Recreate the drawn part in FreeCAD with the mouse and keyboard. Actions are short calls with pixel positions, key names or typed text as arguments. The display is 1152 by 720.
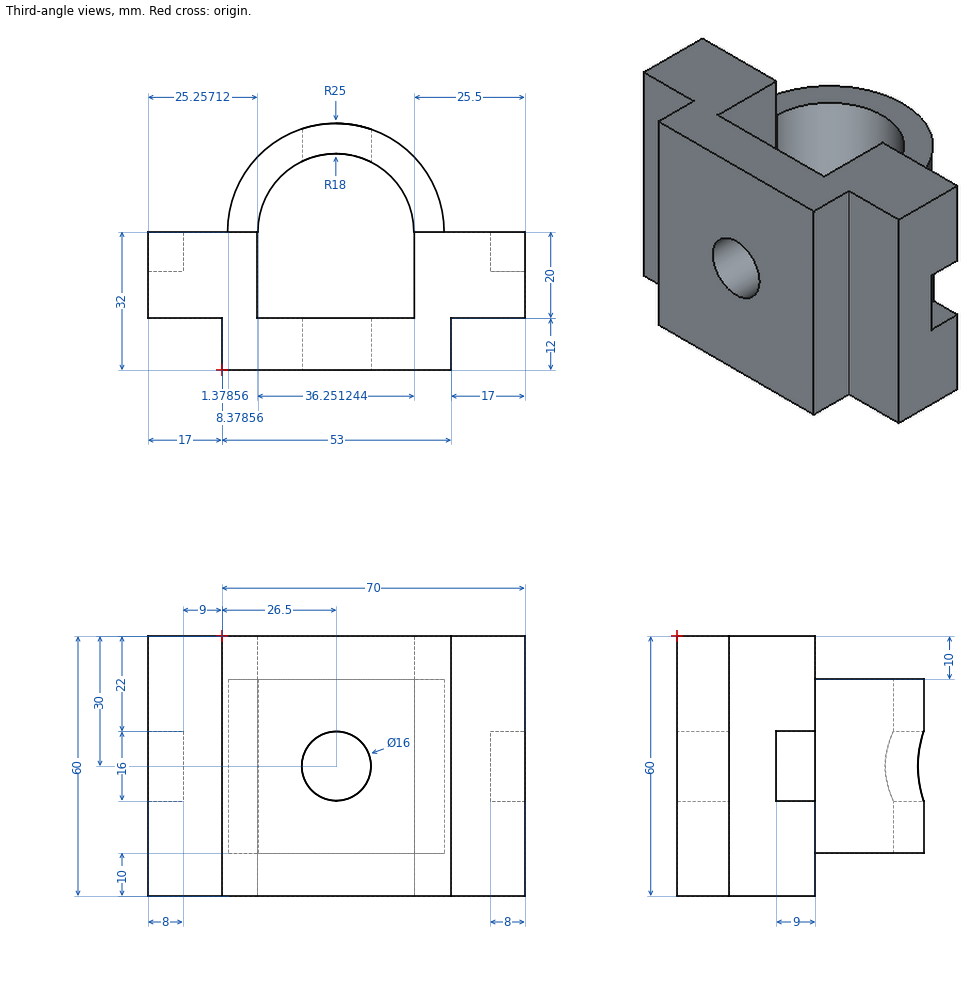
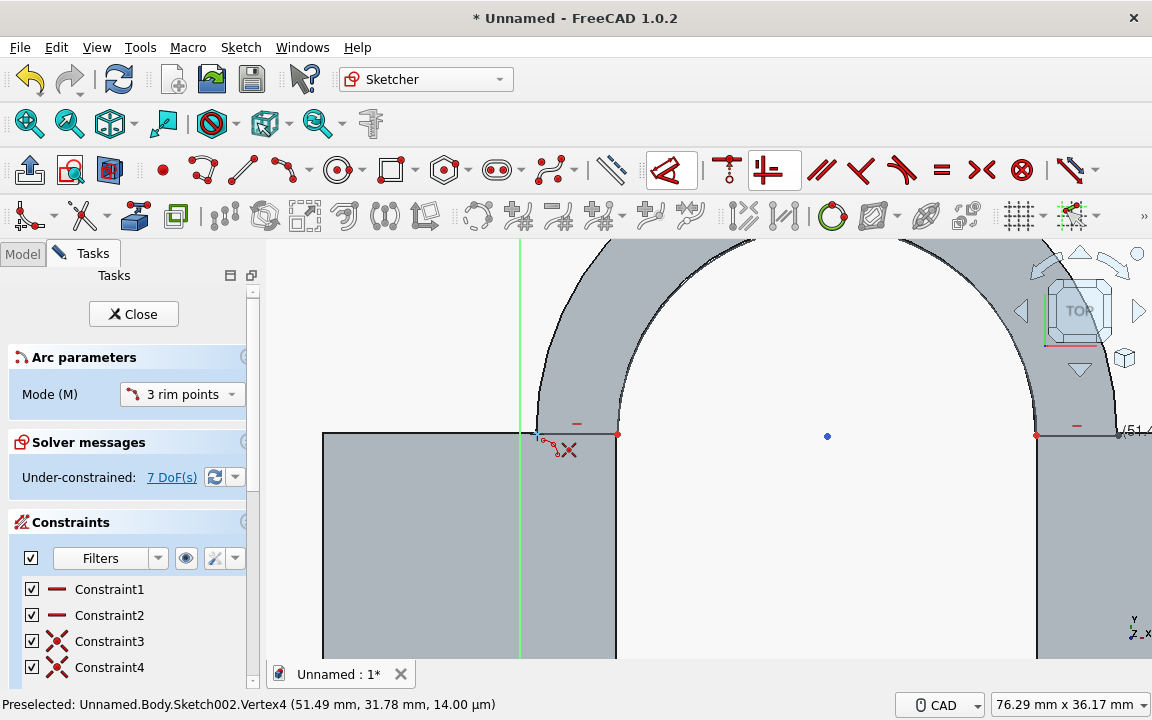
click(537, 434)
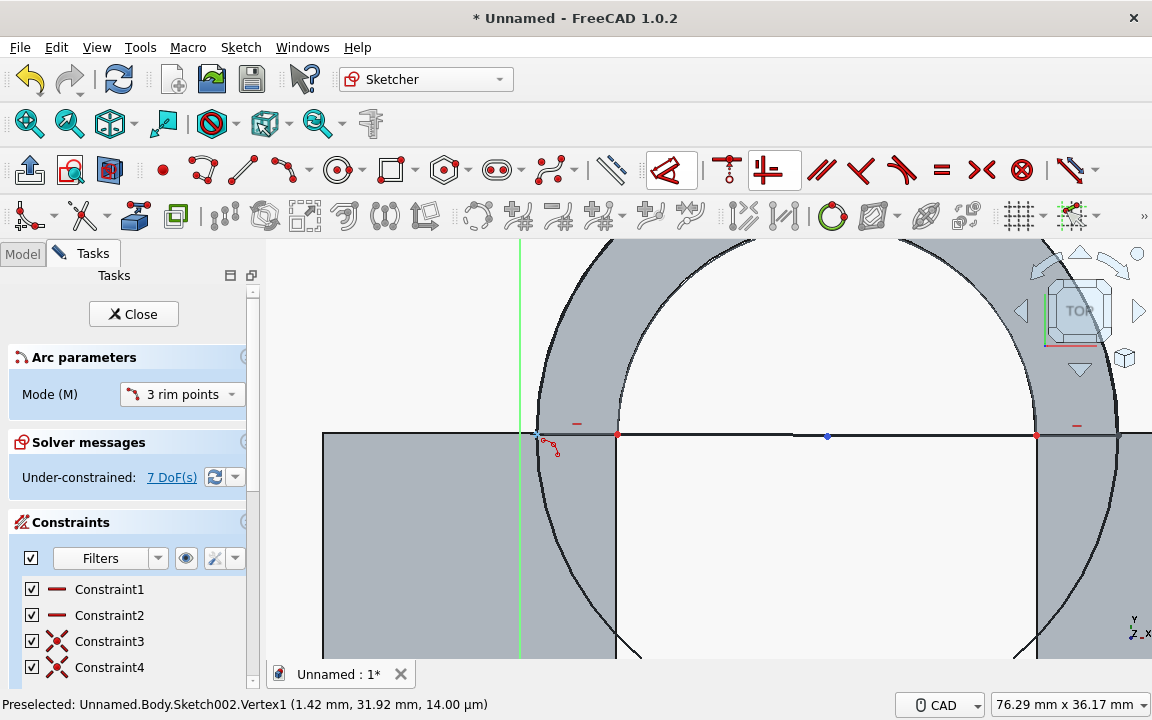
scroll(537, 434, down, 5)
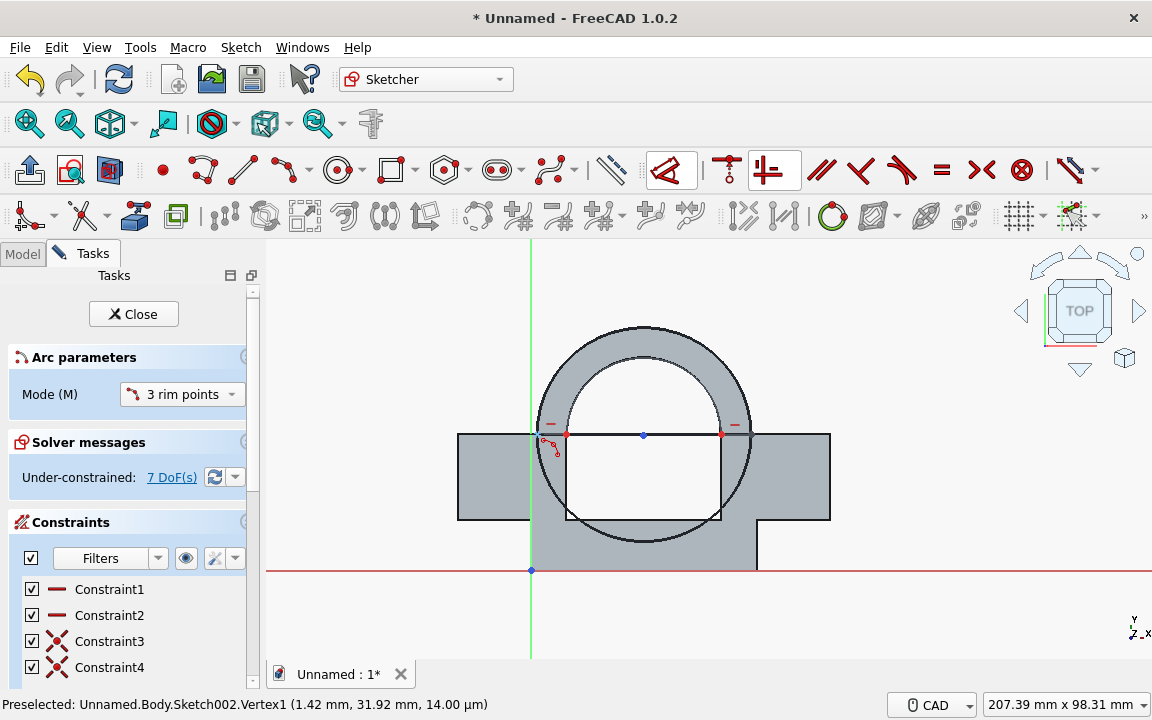
click(644, 327)
key(Escape)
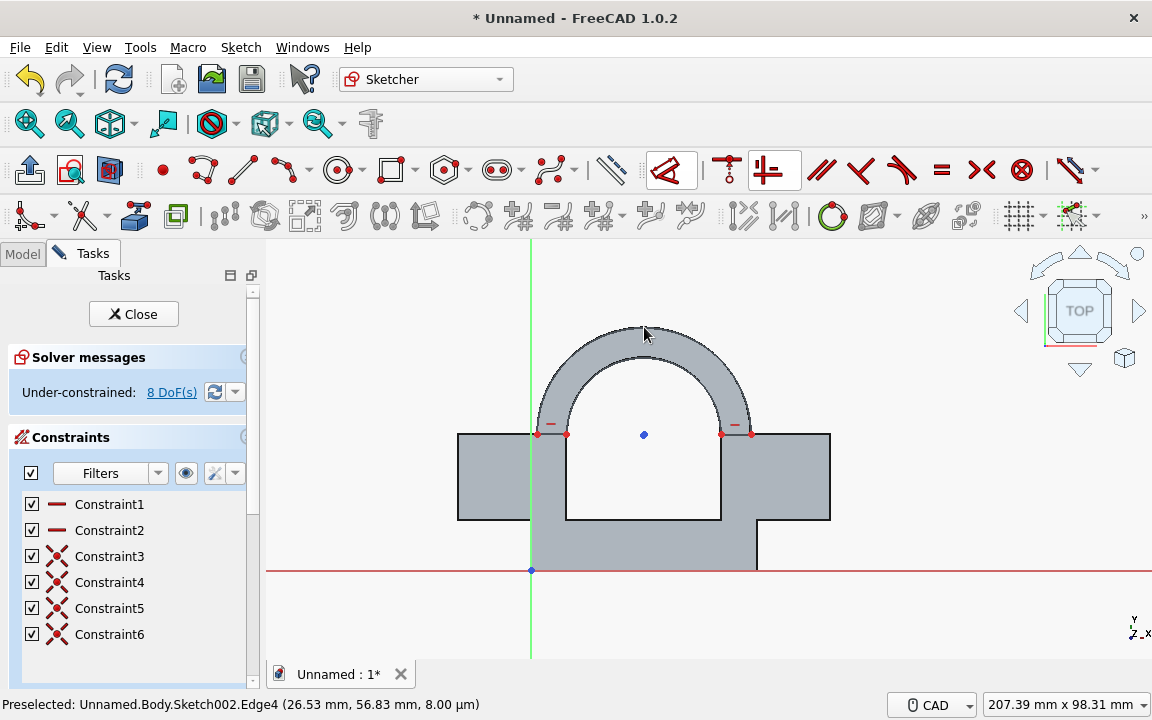
click(689, 373)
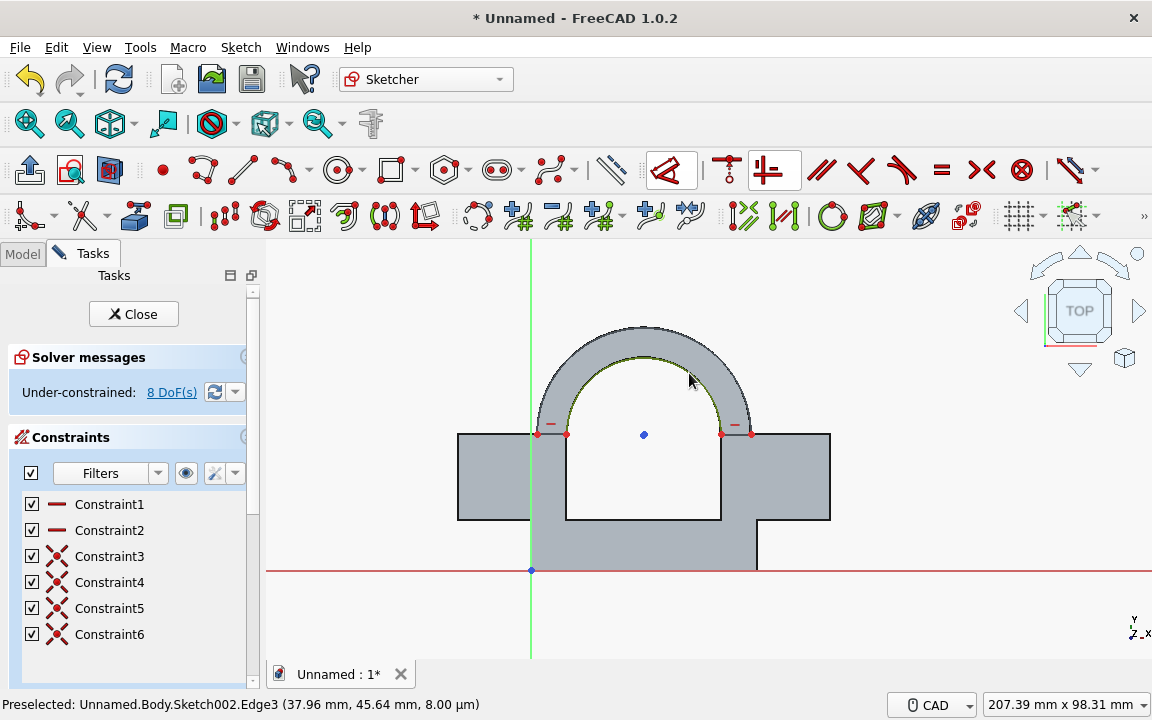
click(707, 349)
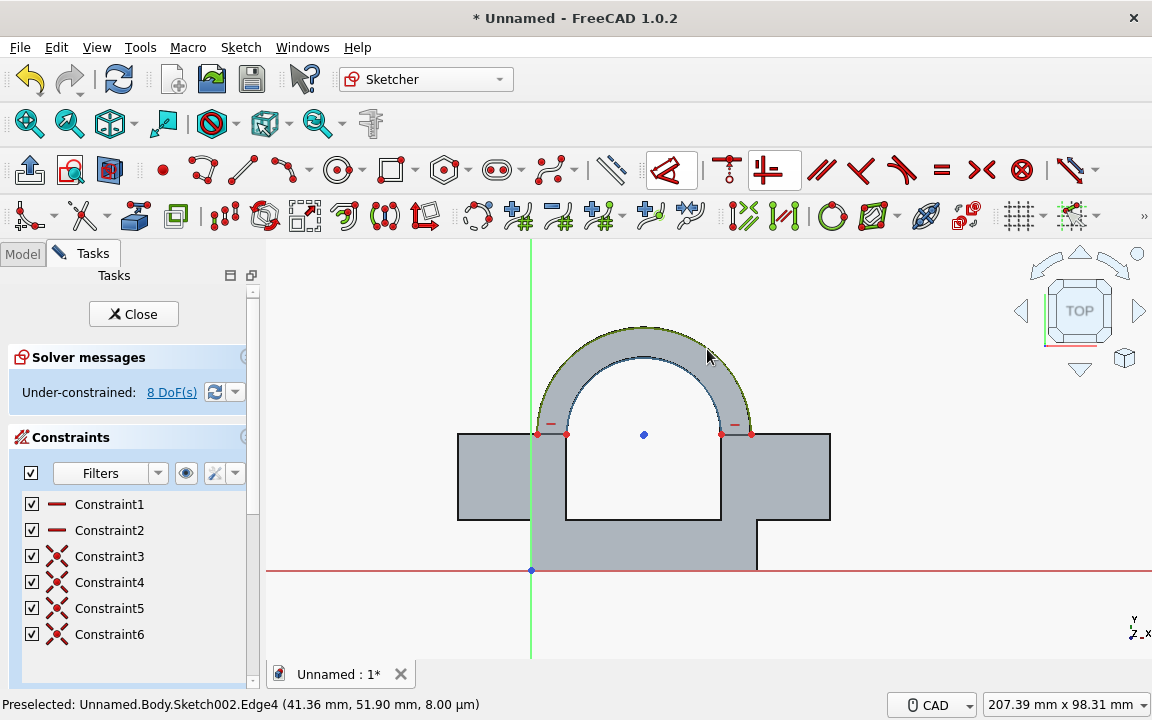
key(c)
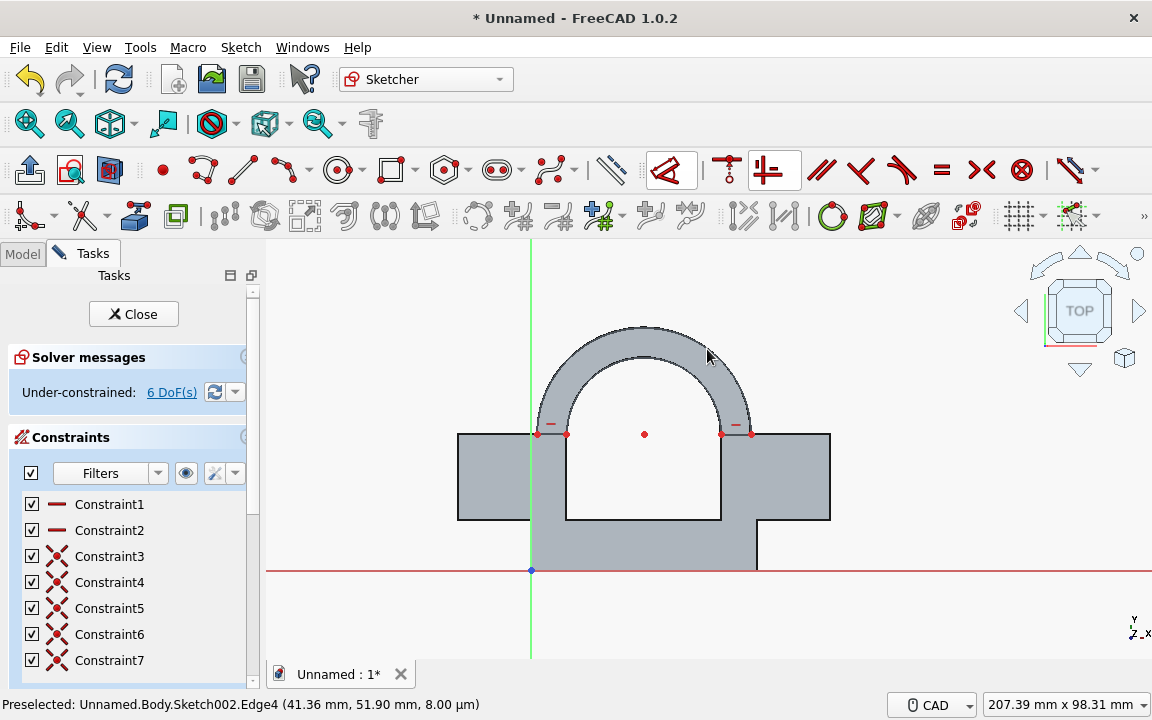
click(690, 373)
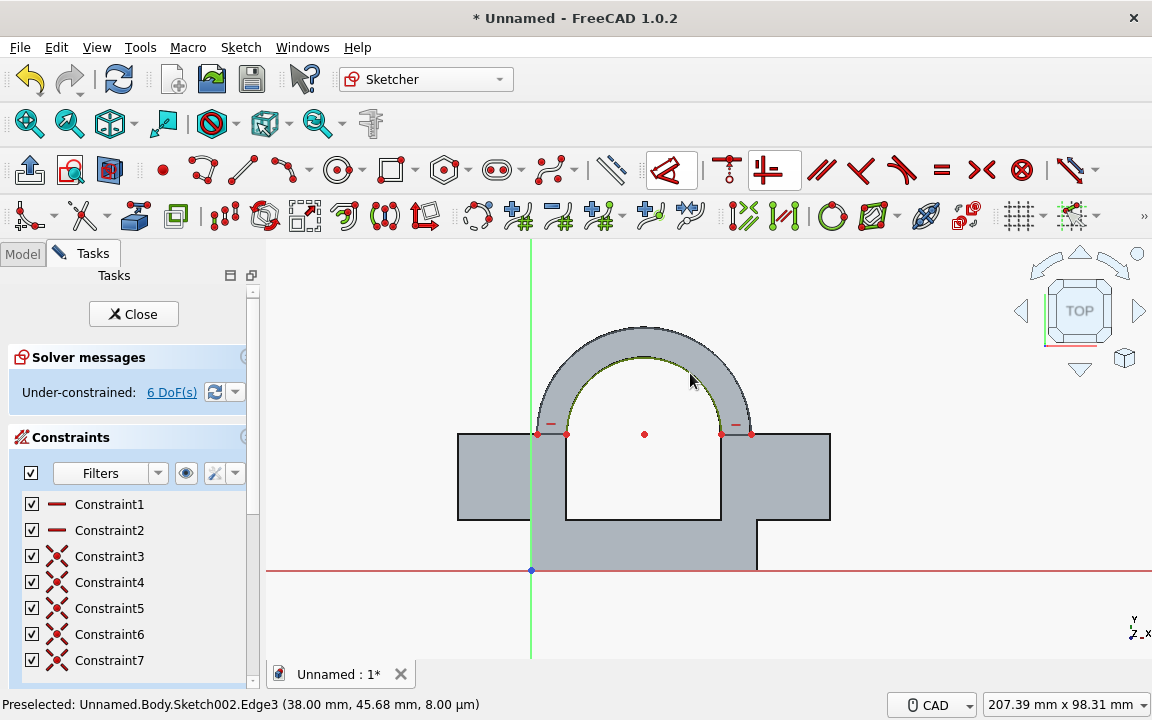
key(k)
key(r)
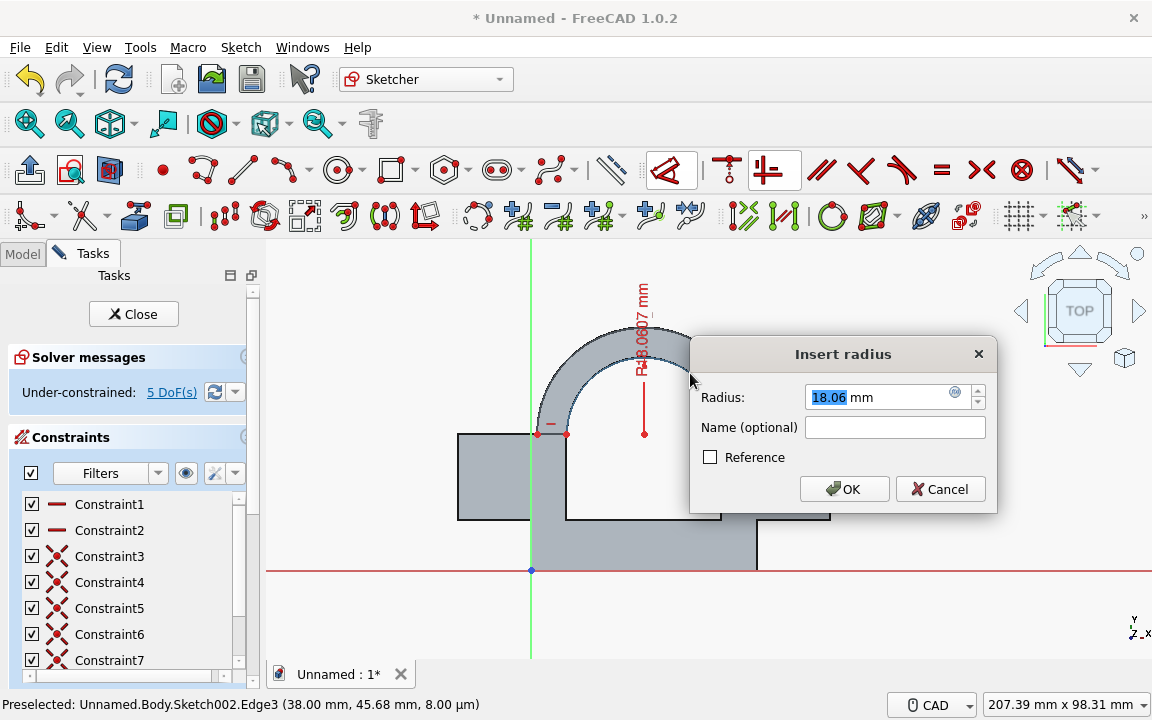
text(18)
key(Return)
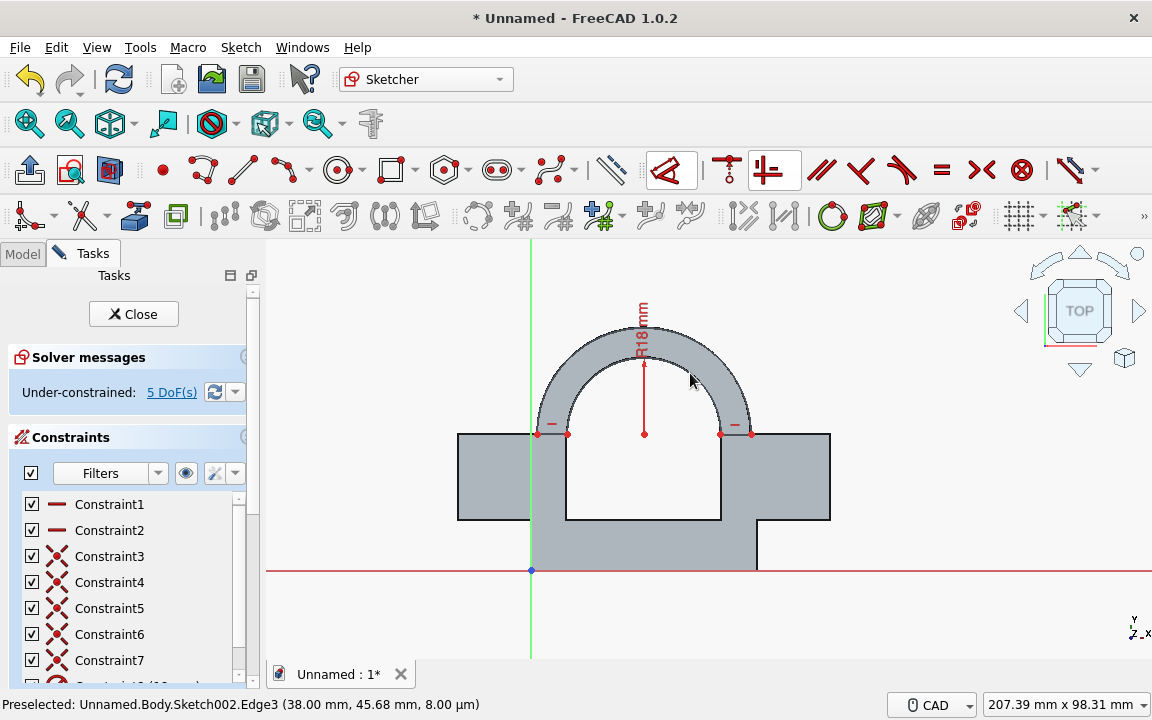
click(707, 349)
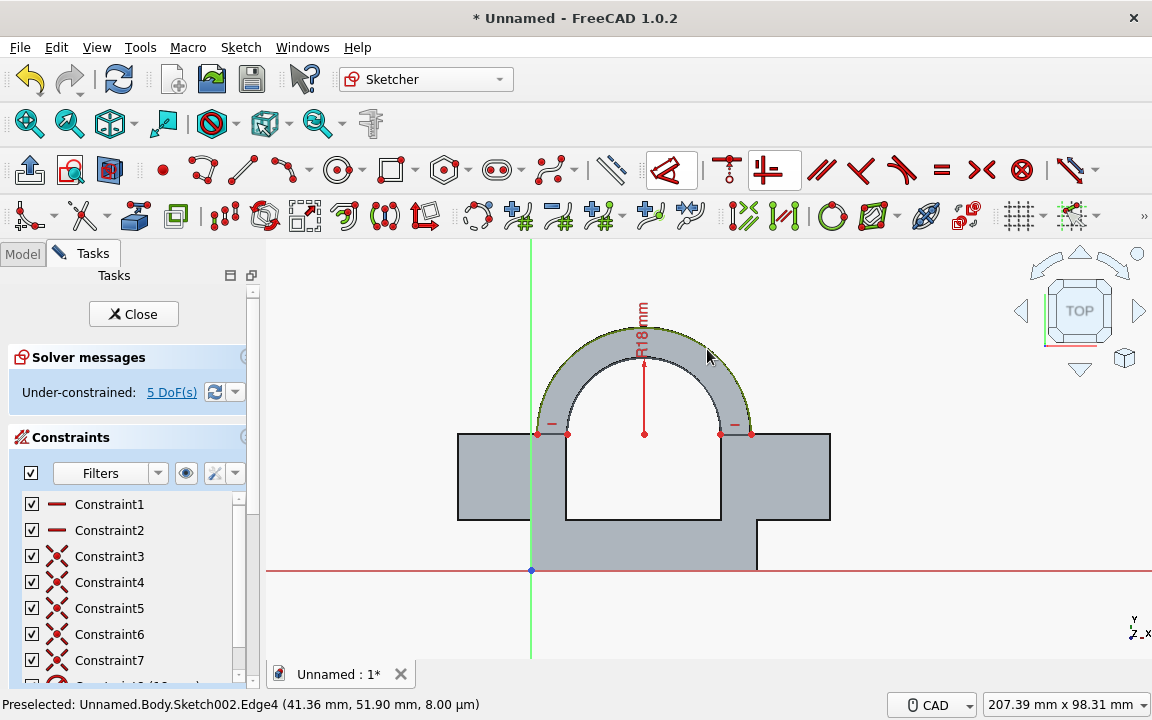
key(k)
key(r)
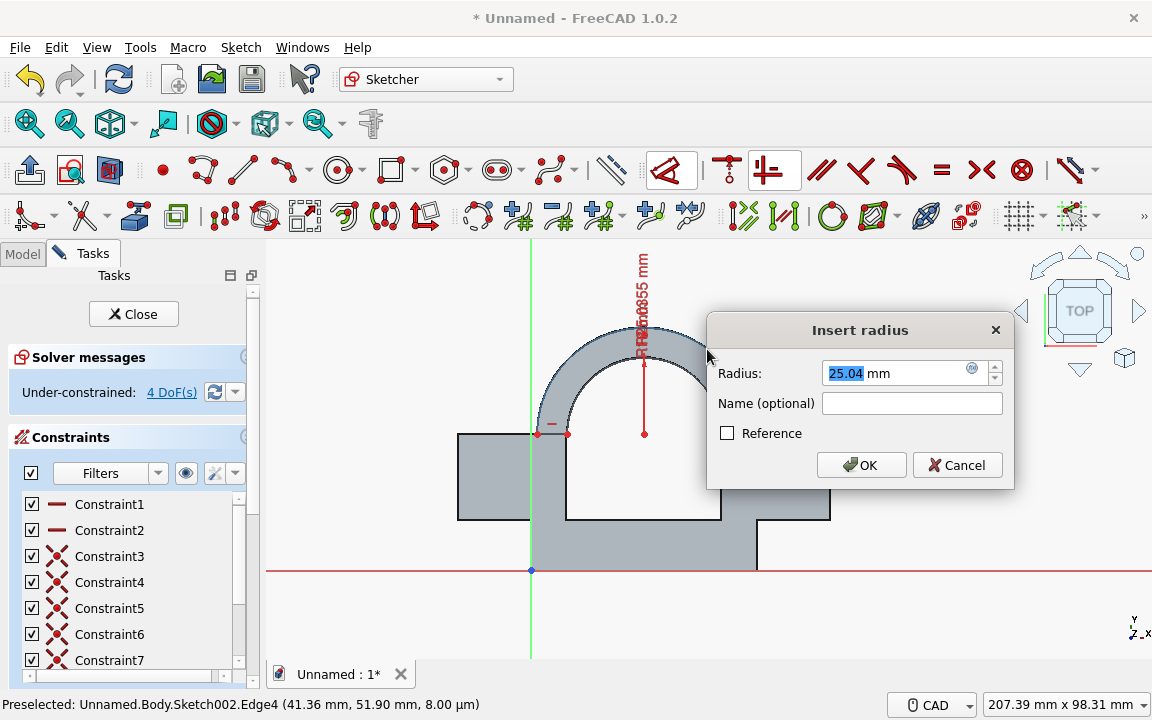
text(25)
key(Return)